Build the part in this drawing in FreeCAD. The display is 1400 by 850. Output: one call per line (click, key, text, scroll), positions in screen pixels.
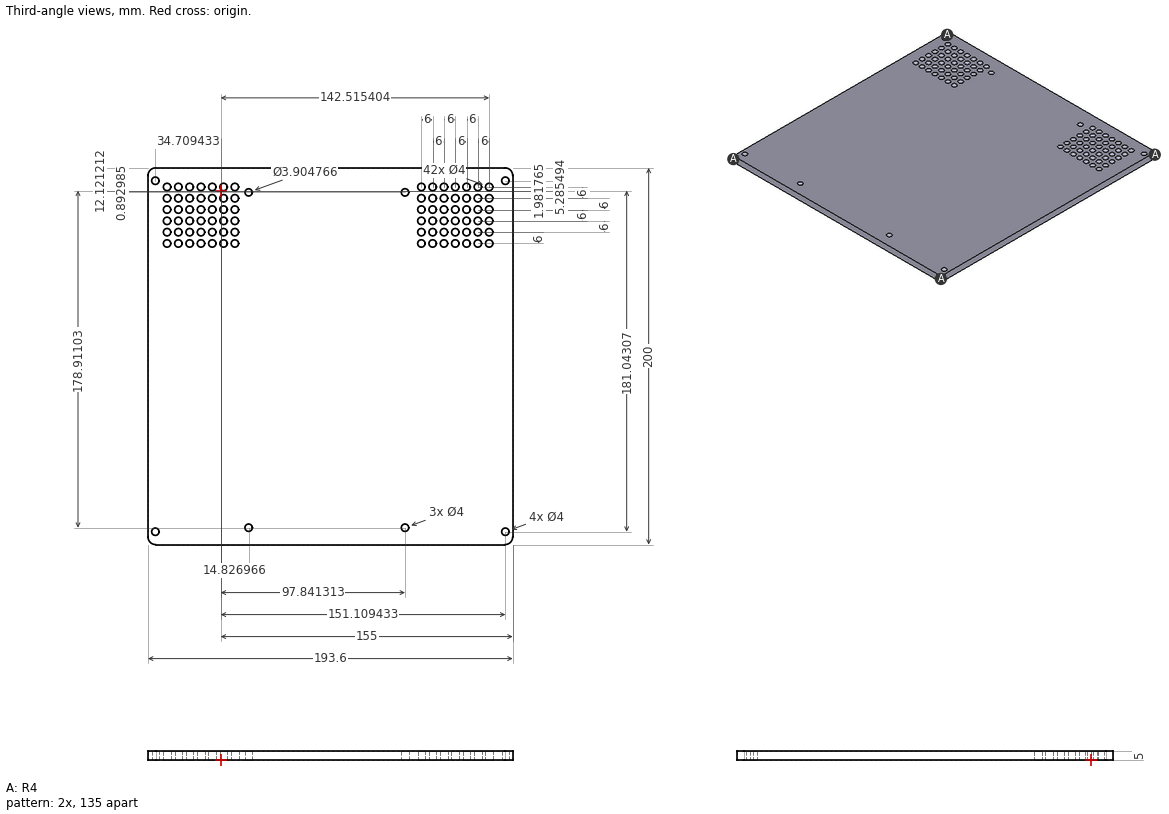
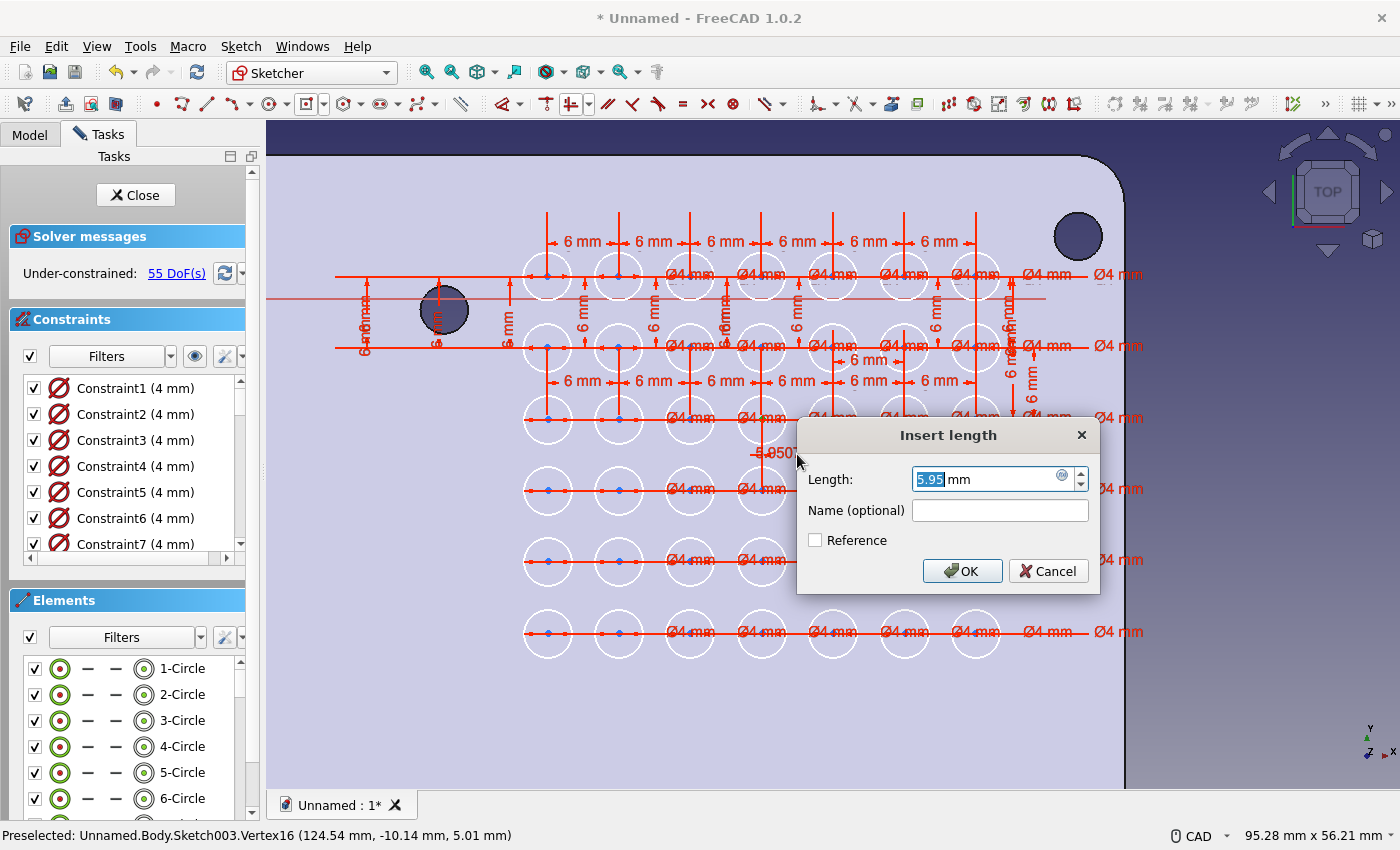
text(6)
key(Return)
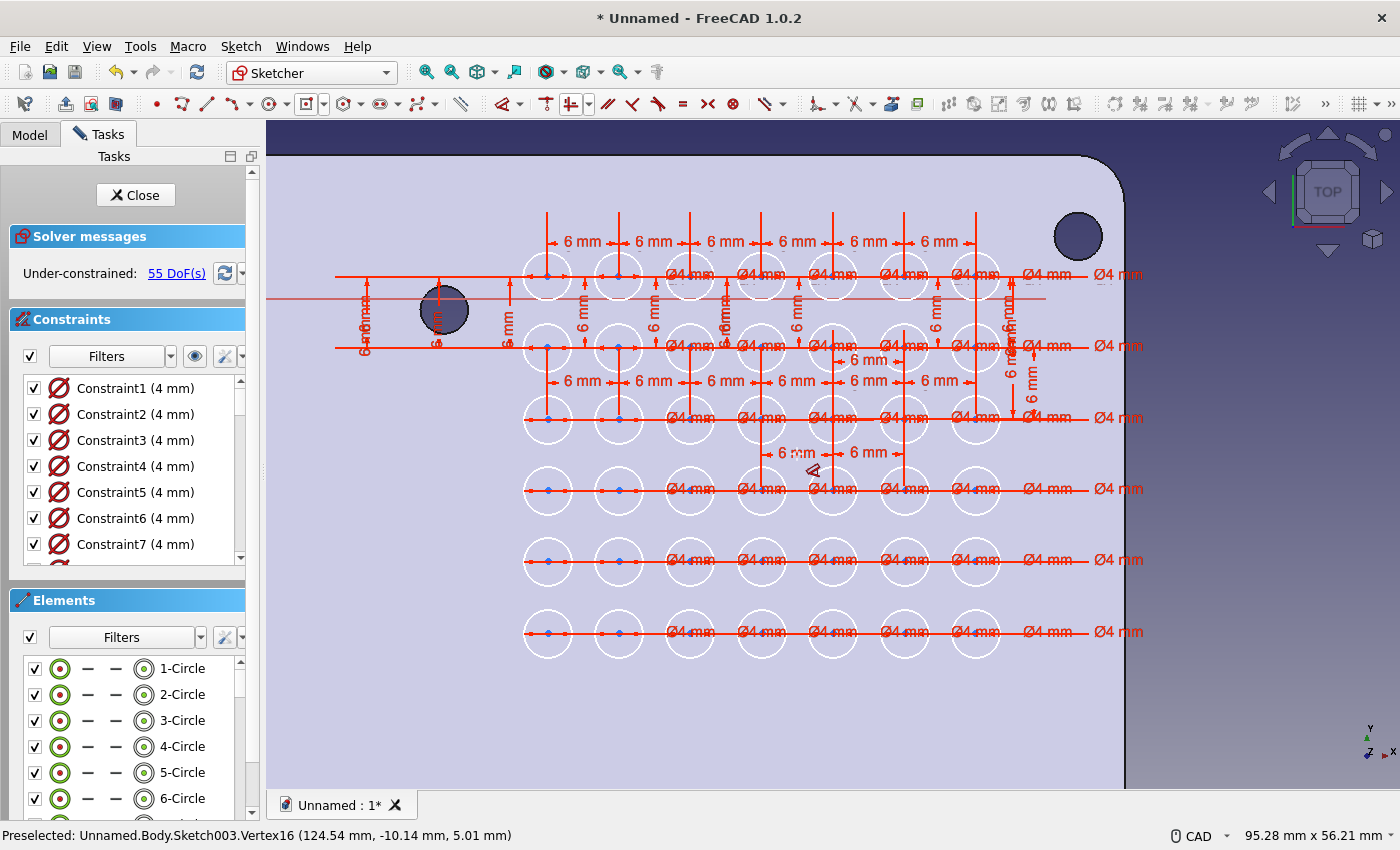
click(761, 348)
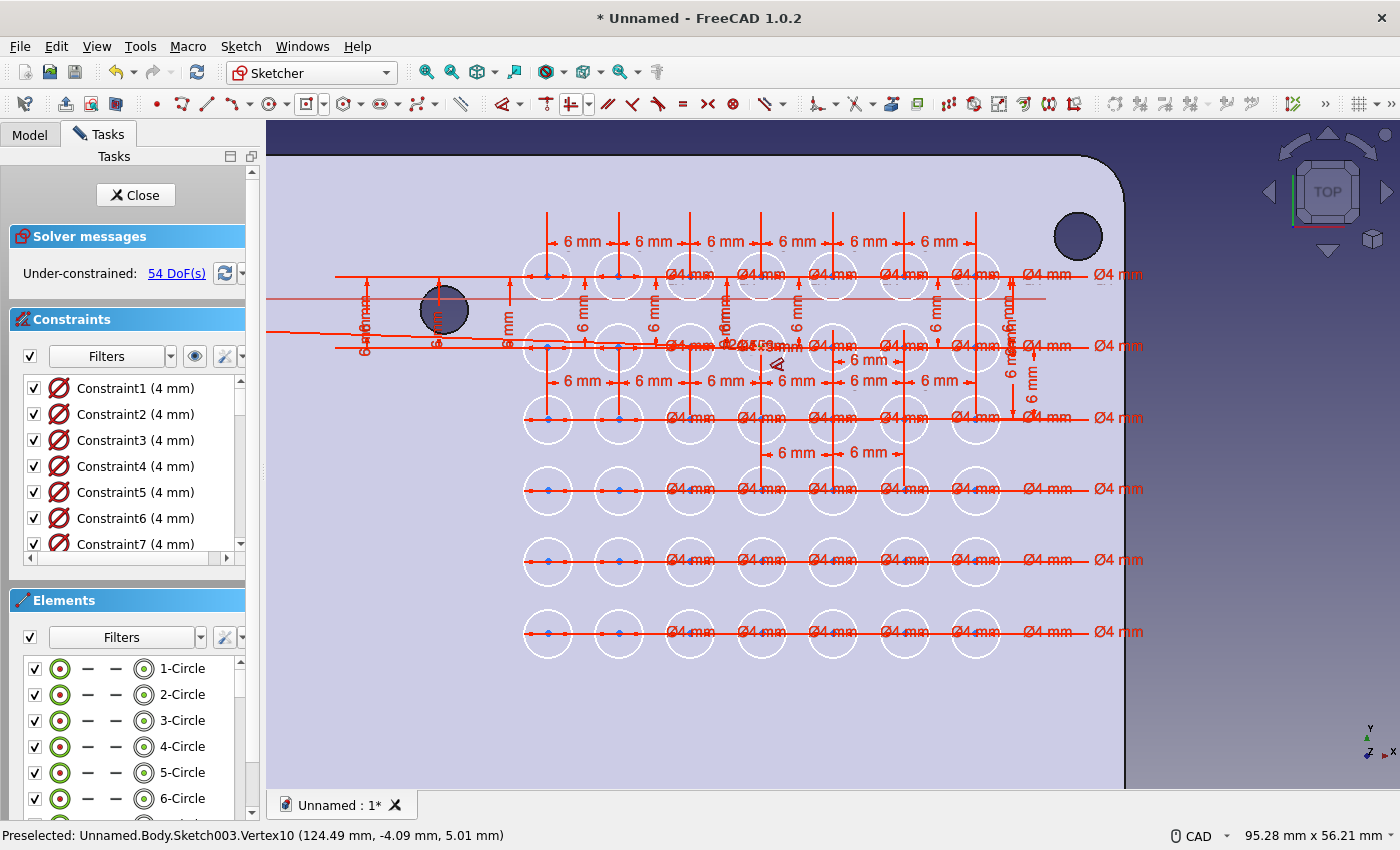
click(761, 420)
click(727, 367)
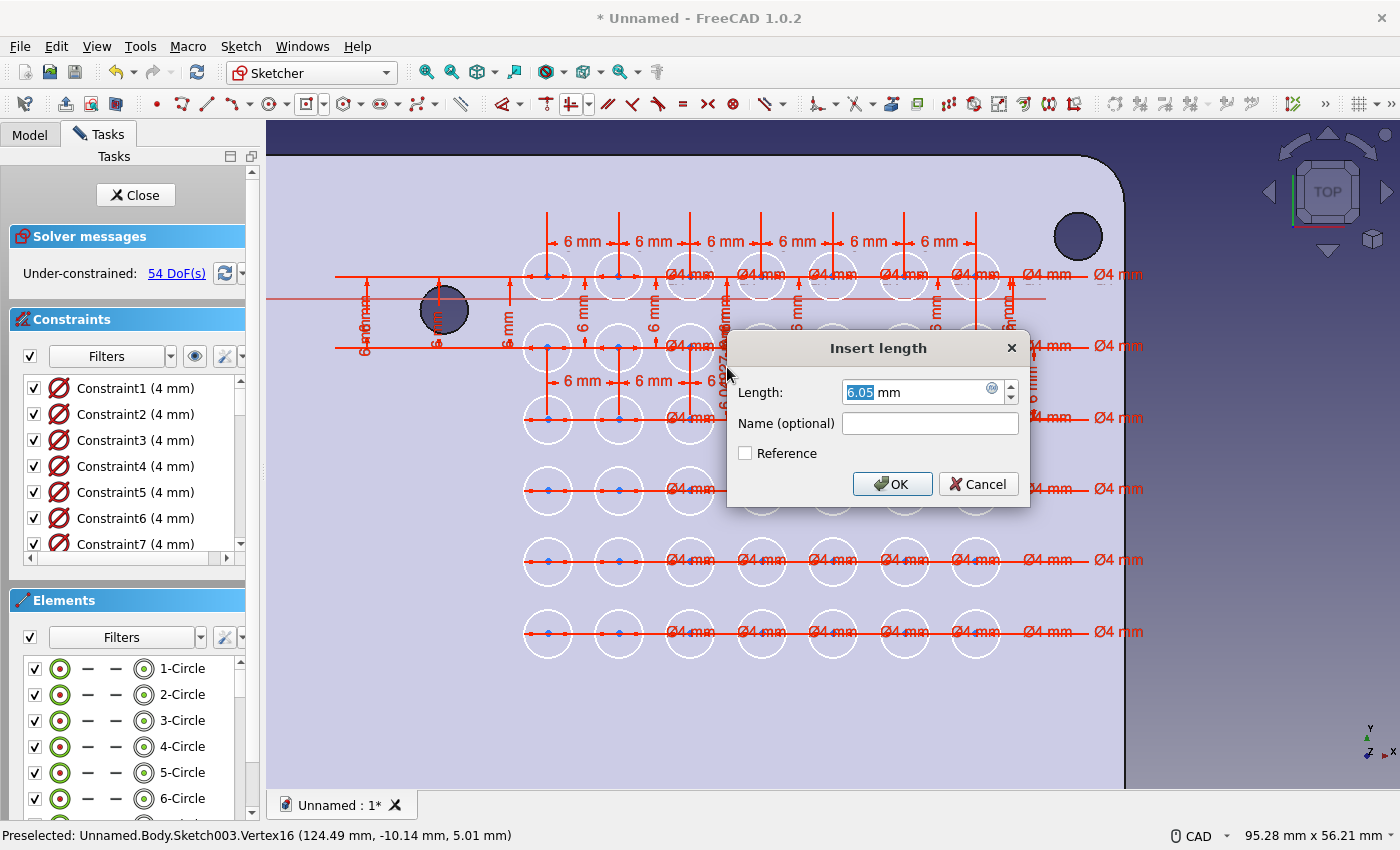
text(6)
key(Return)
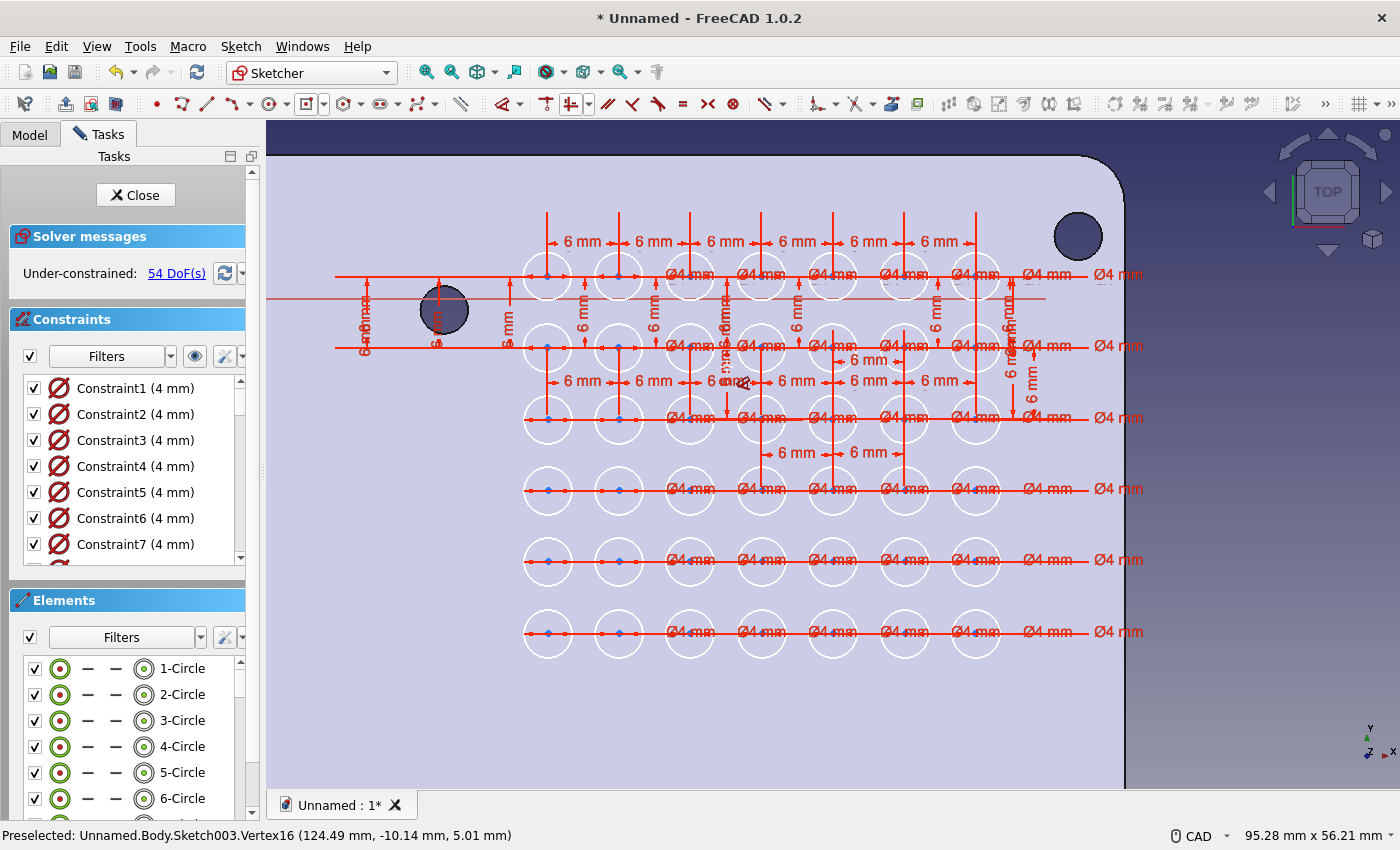
click(761, 419)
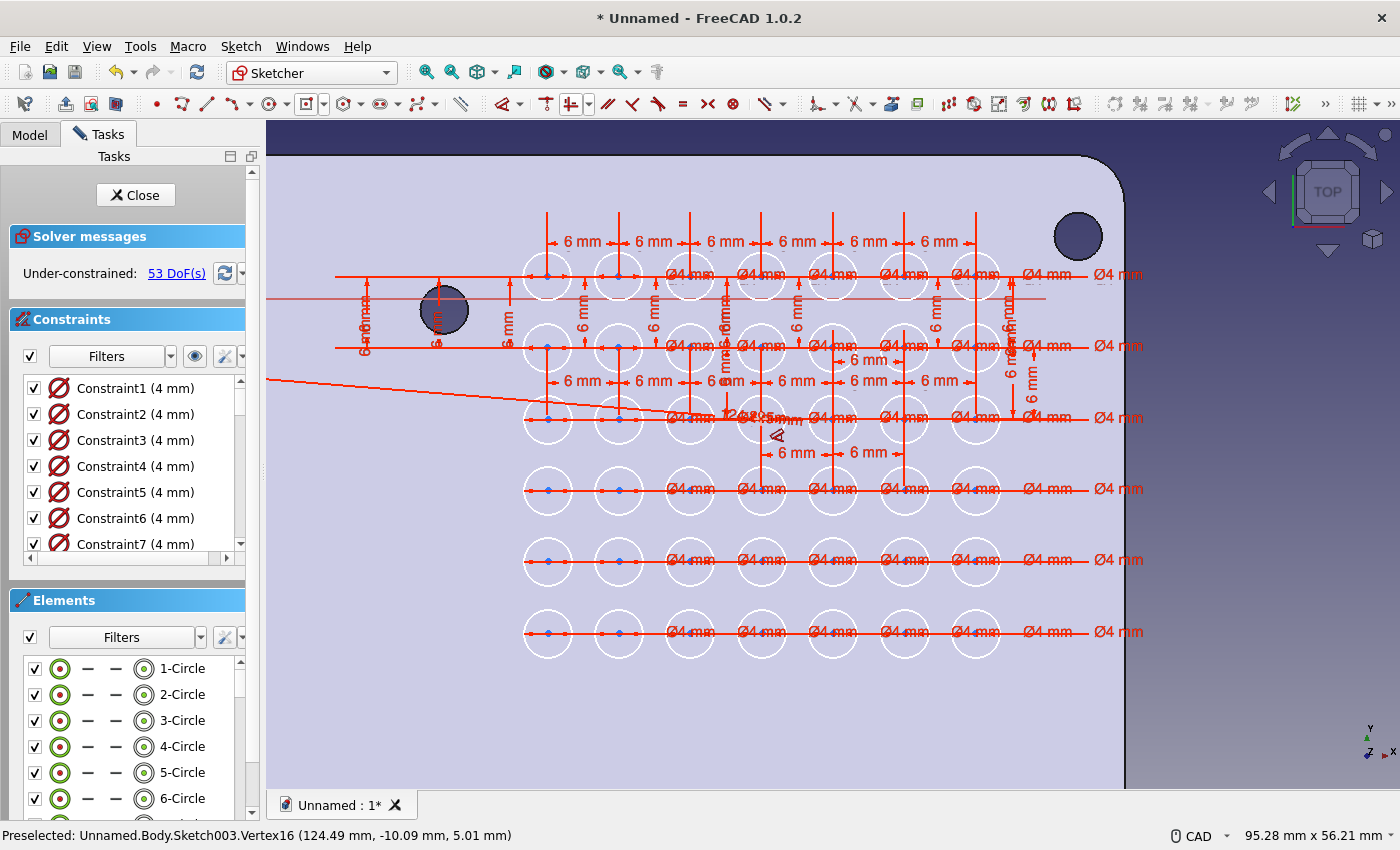
click(690, 420)
click(726, 454)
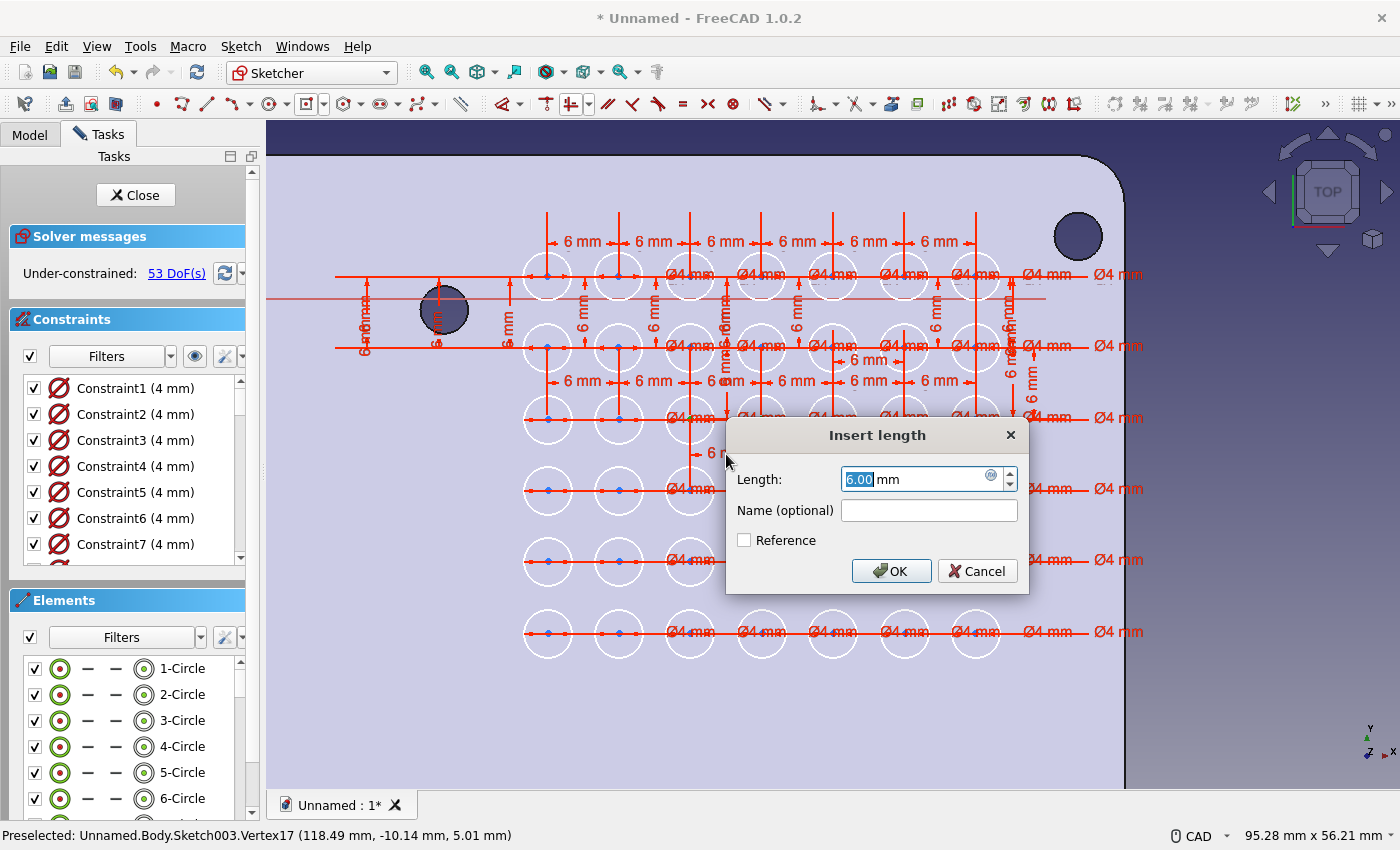
text(6)
key(Return)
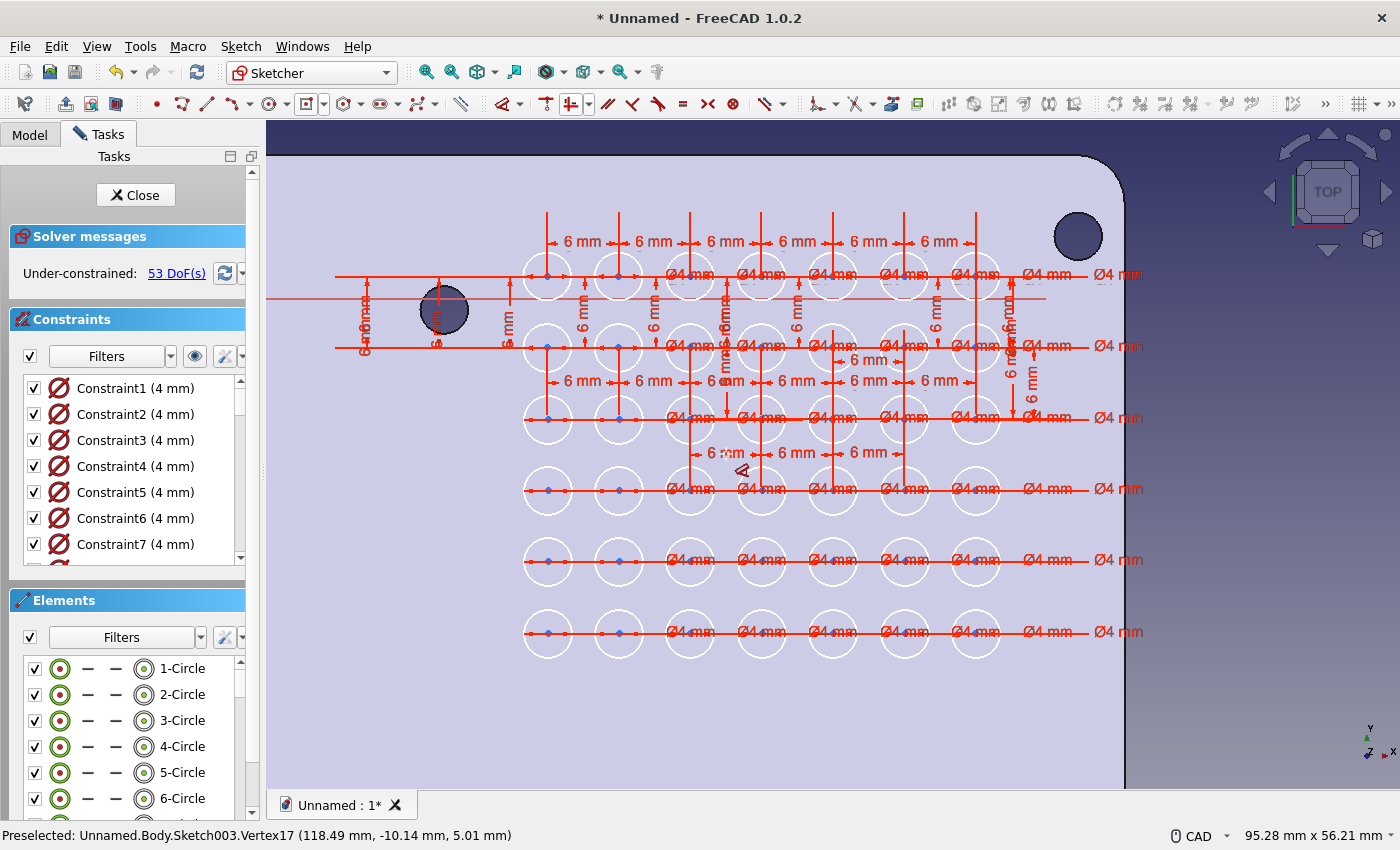
click(690, 348)